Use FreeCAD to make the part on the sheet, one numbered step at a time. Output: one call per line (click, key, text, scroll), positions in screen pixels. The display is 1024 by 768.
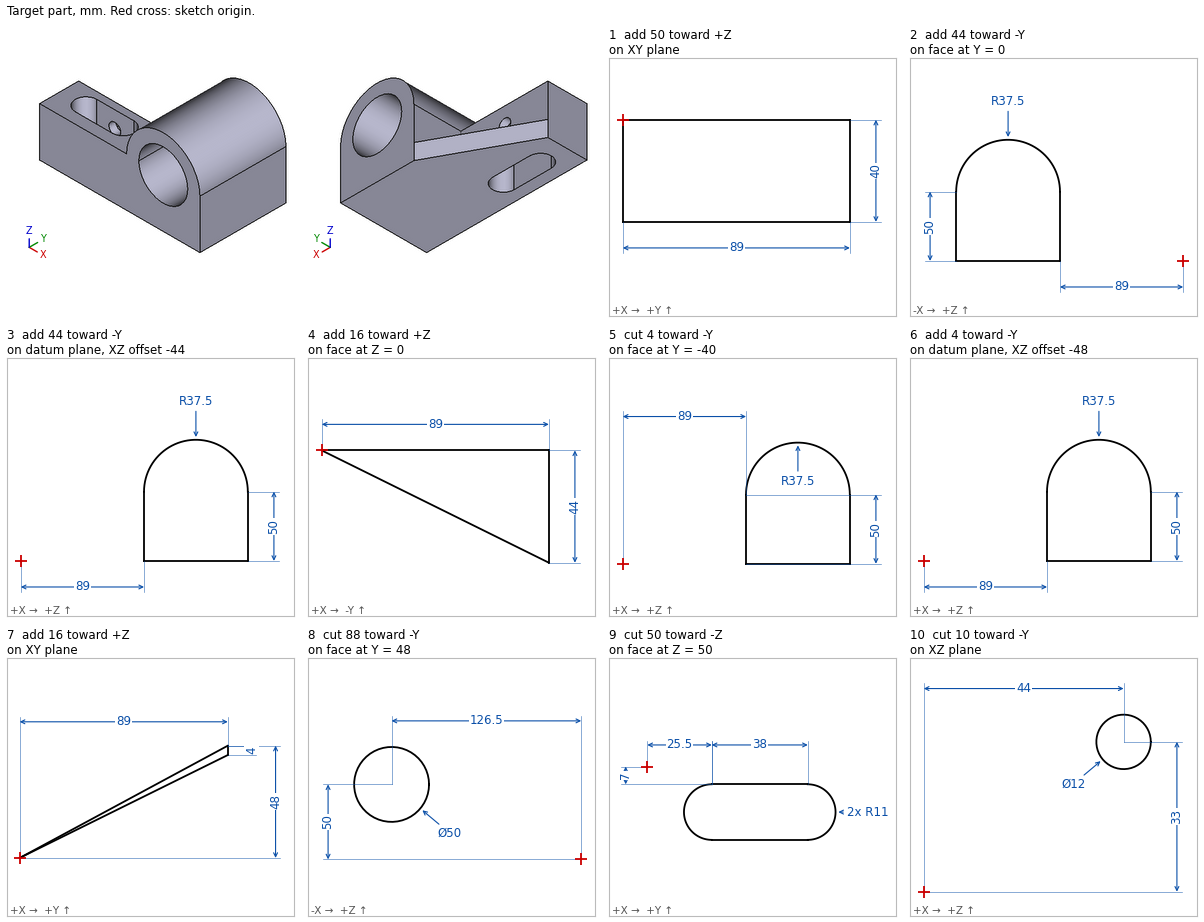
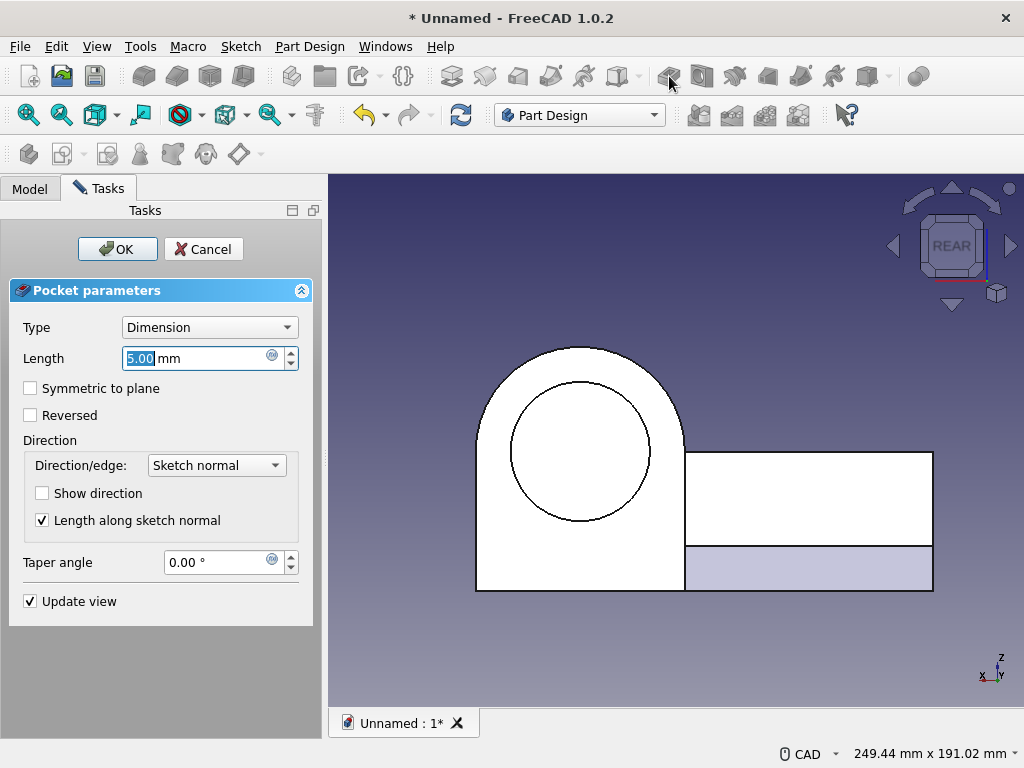
text(88)
key(Tab)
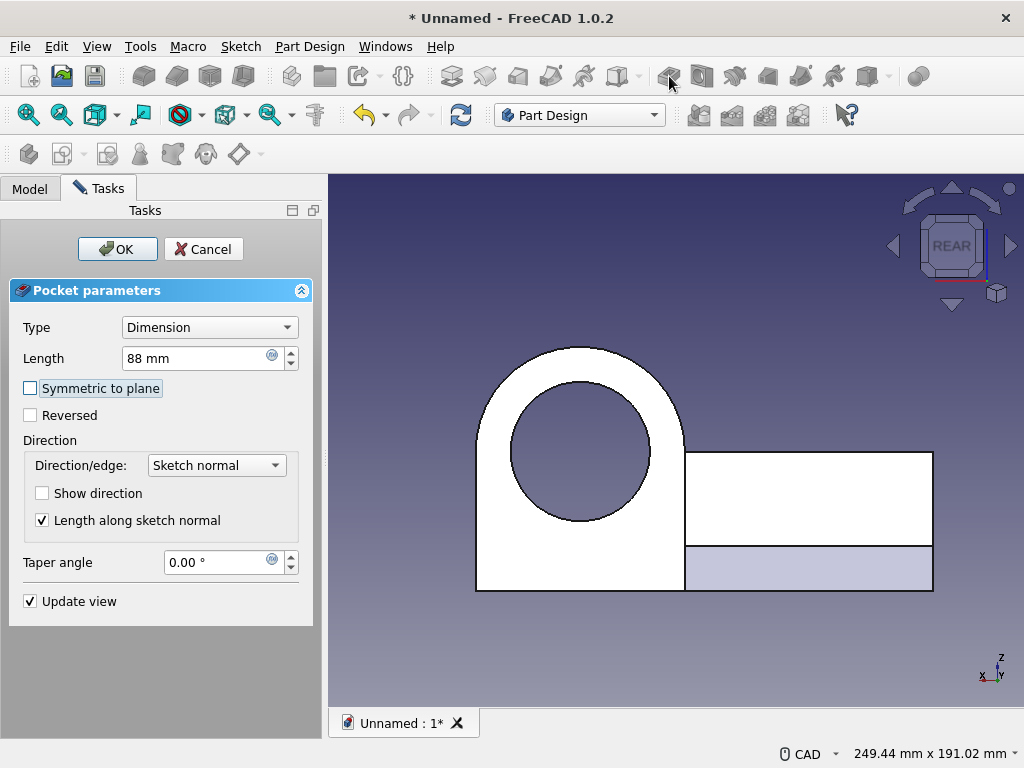
click(118, 249)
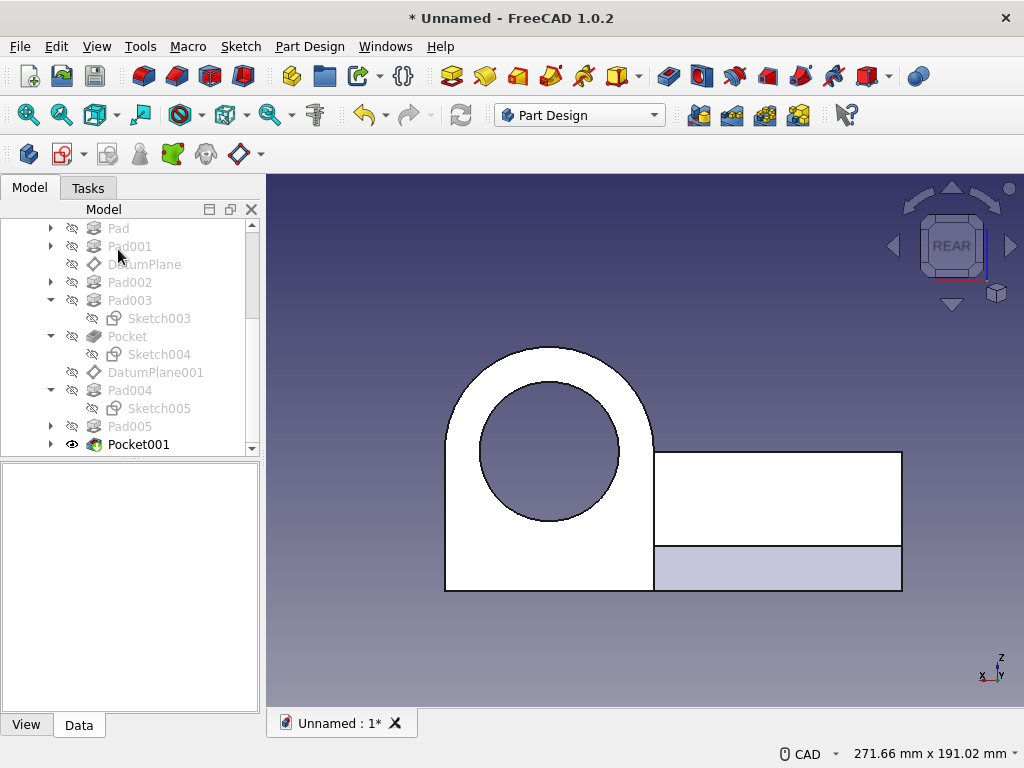
key(0)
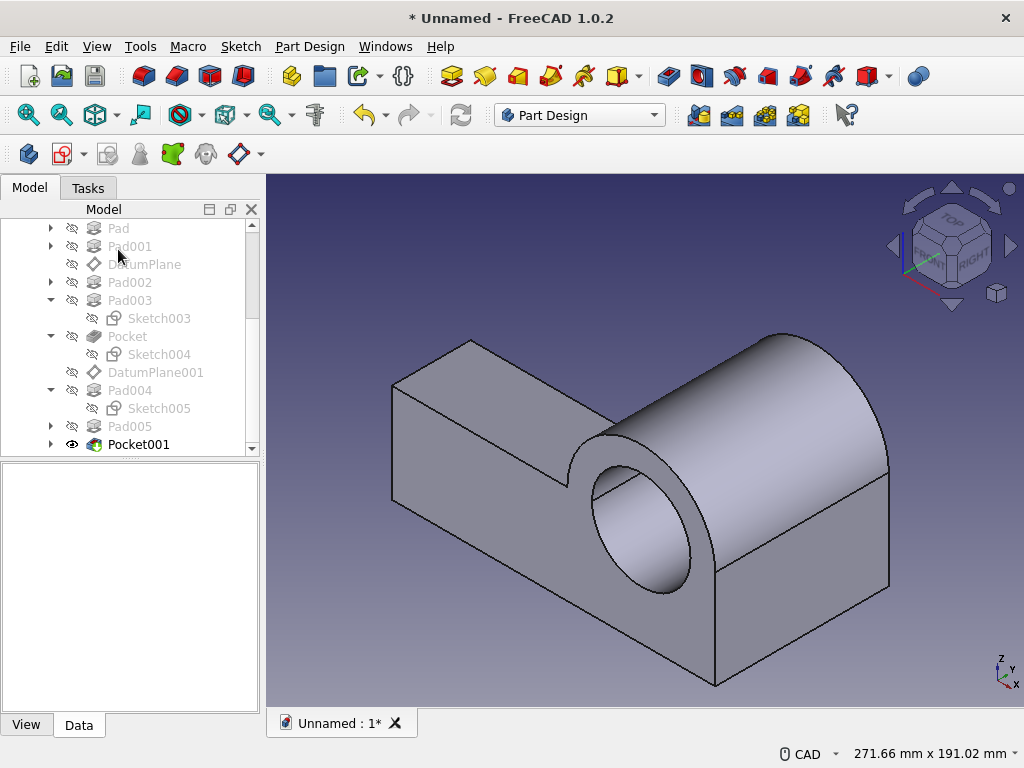
click(544, 427)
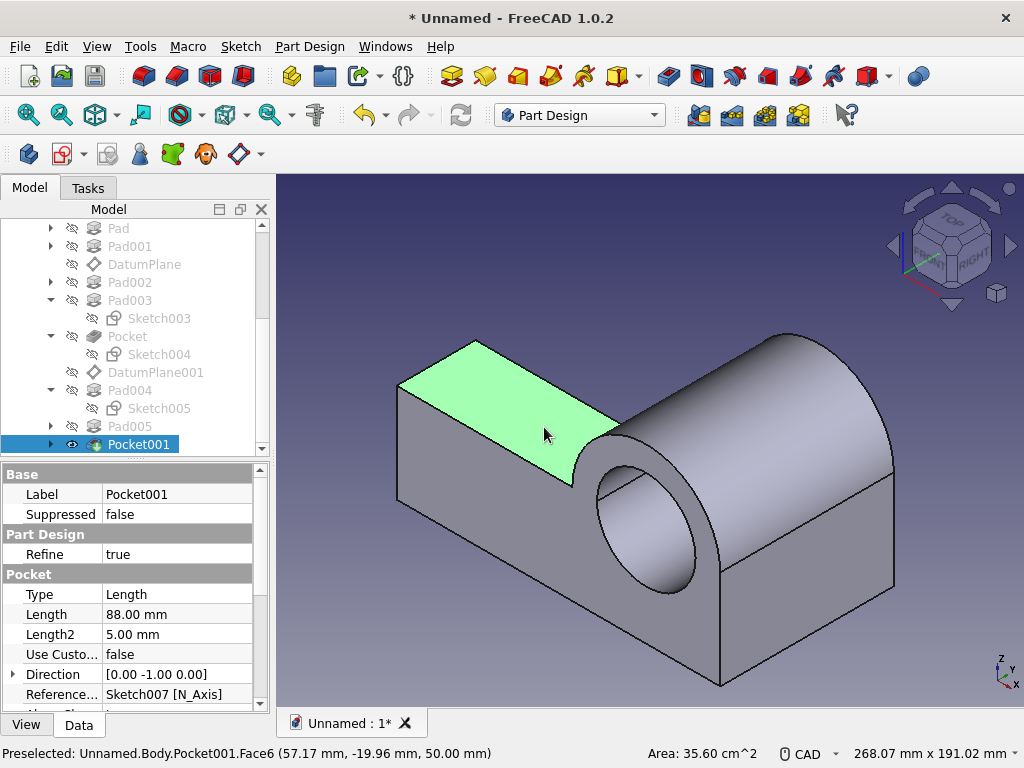
click(62, 154)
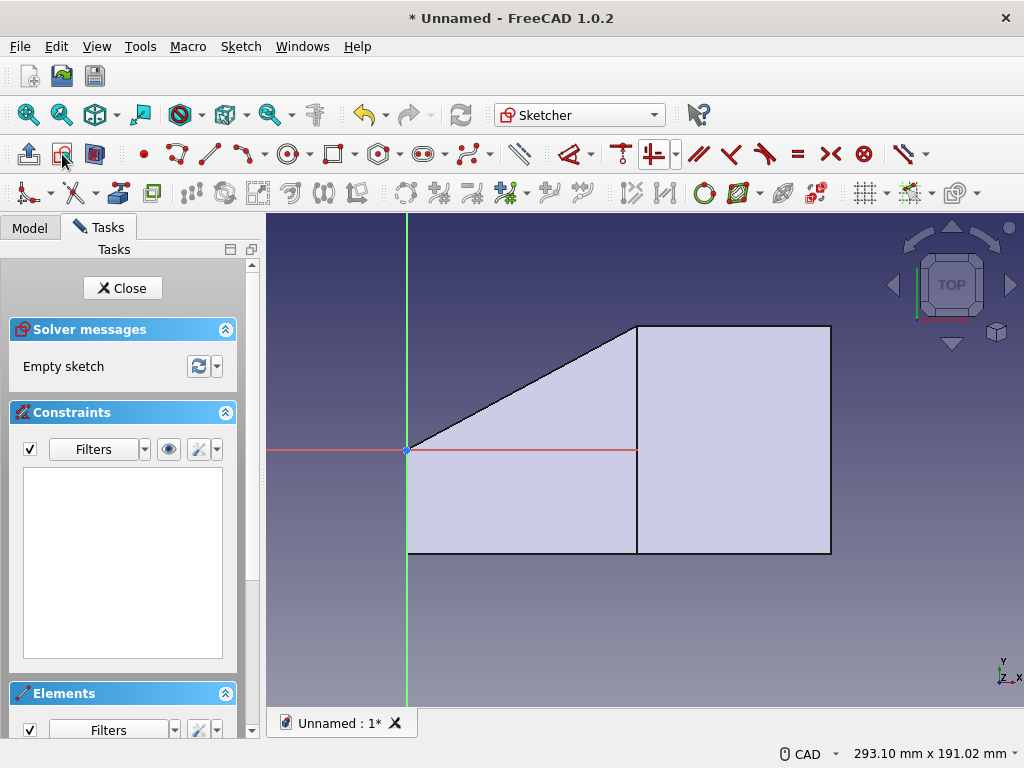
click(95, 154)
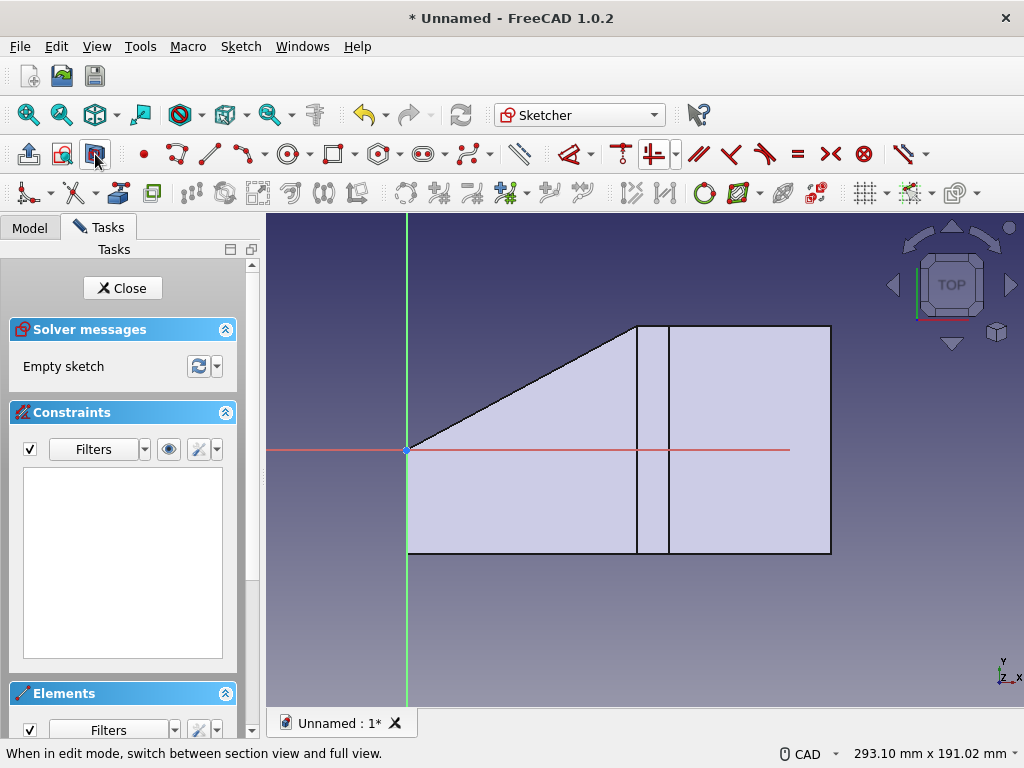
scroll(443, 510, up, 4)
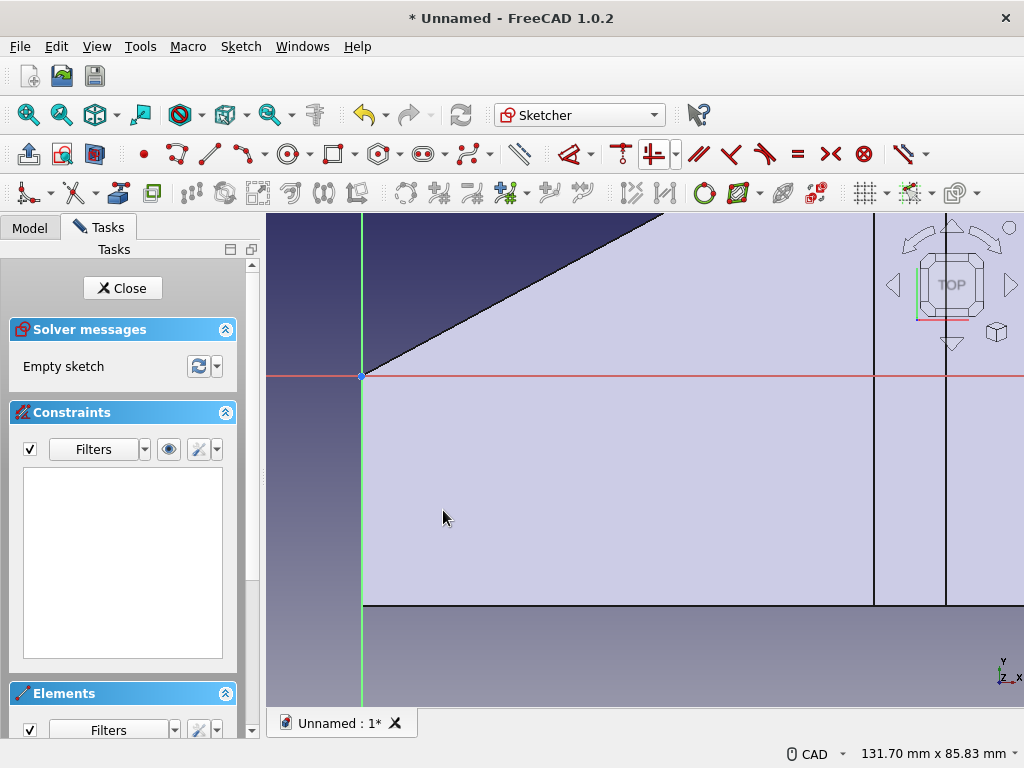
click(422, 154)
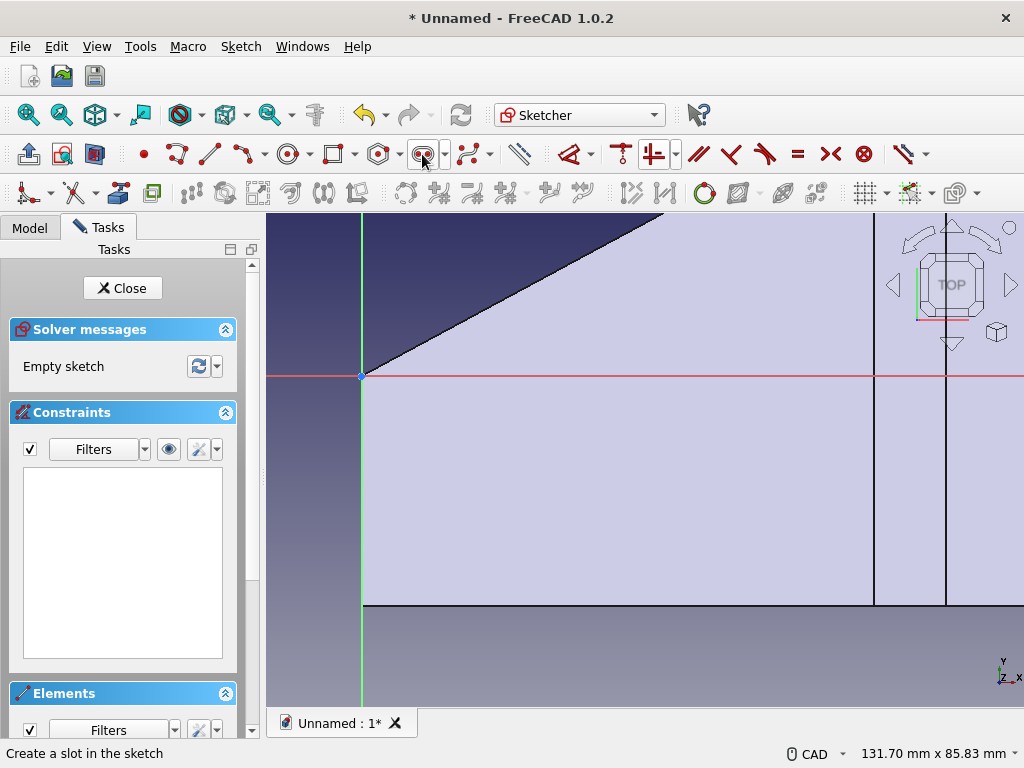
click(508, 480)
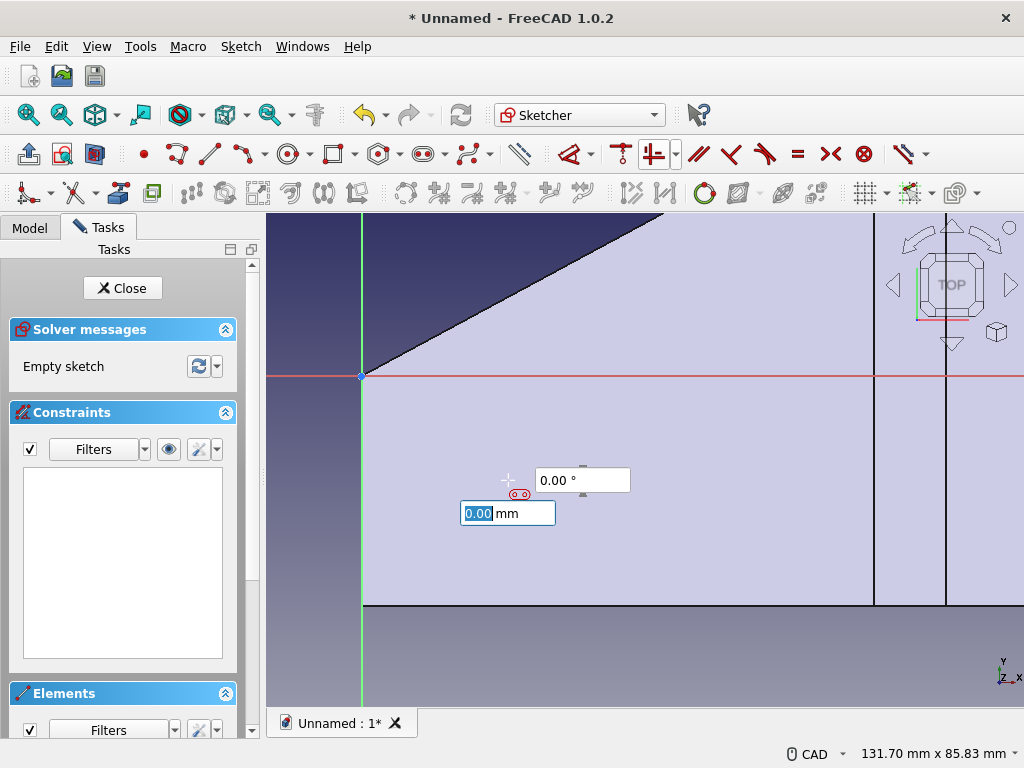
click(727, 480)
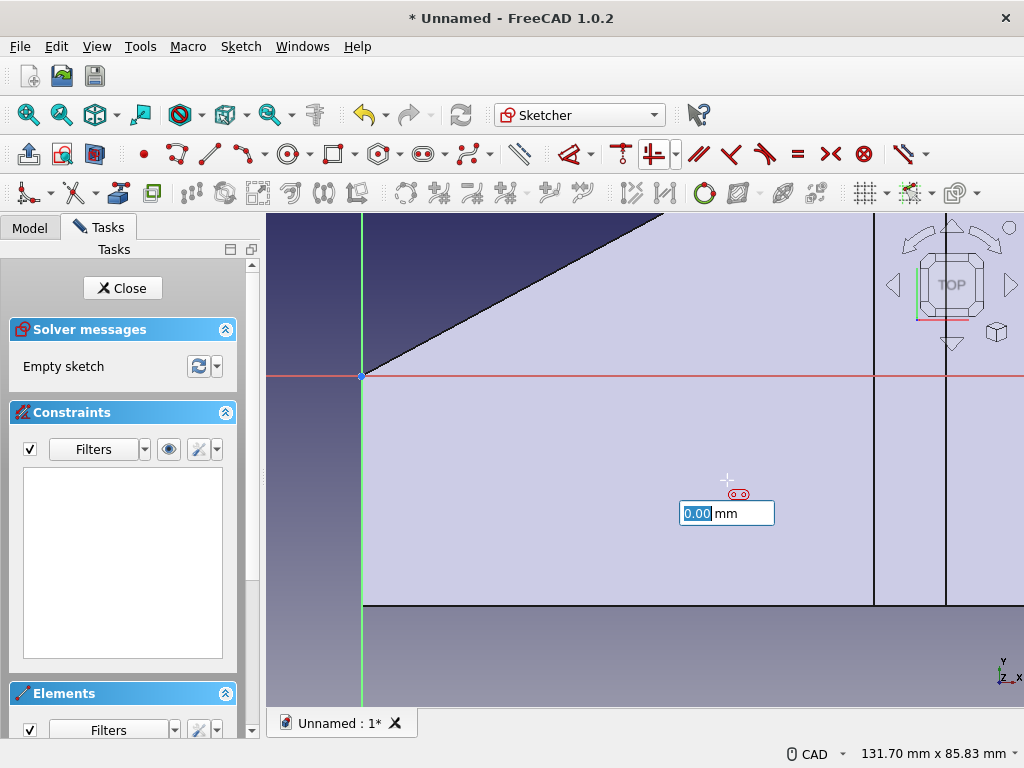
click(618, 543)
key(Escape)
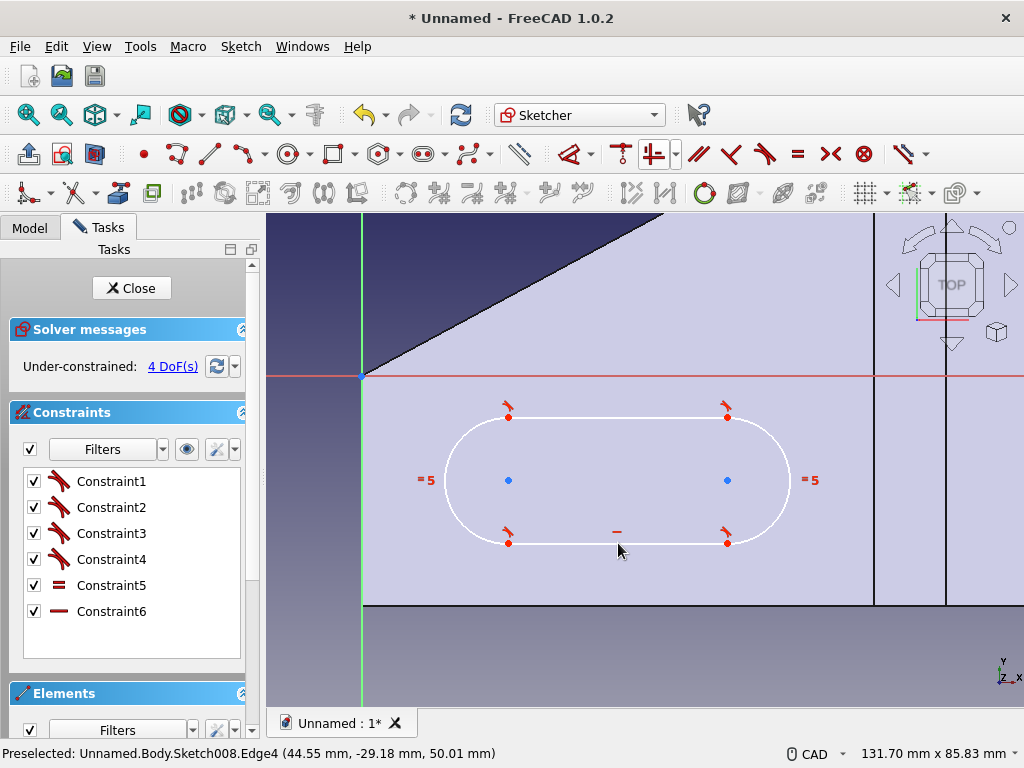
click(568, 154)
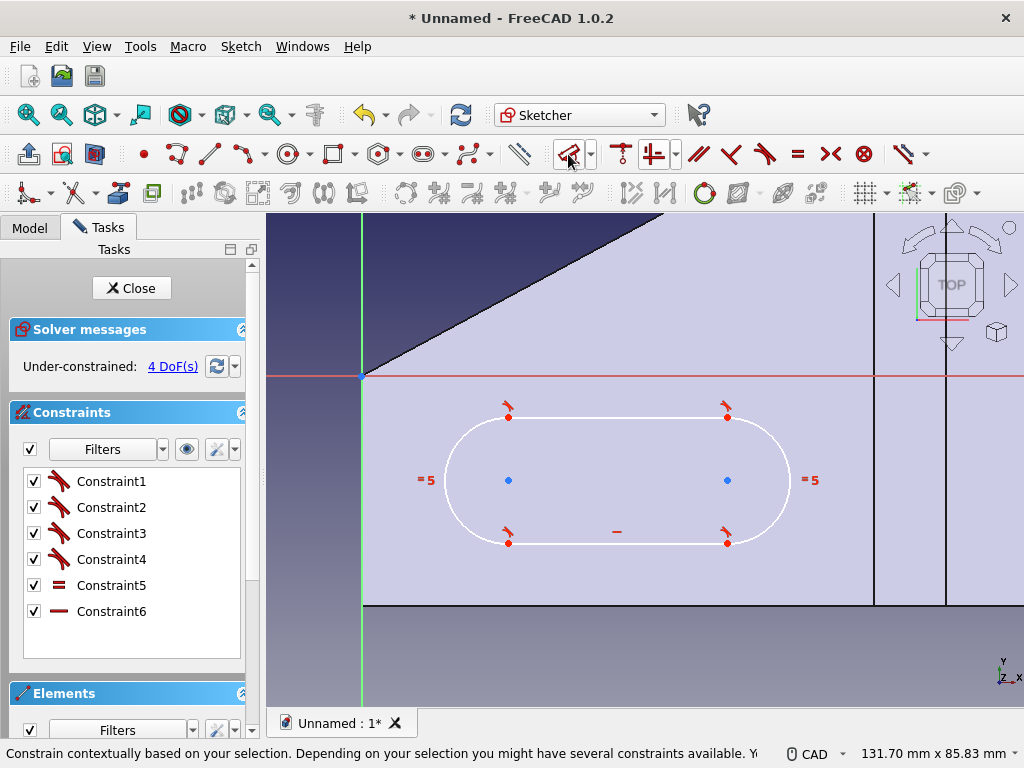
click(457, 444)
click(431, 425)